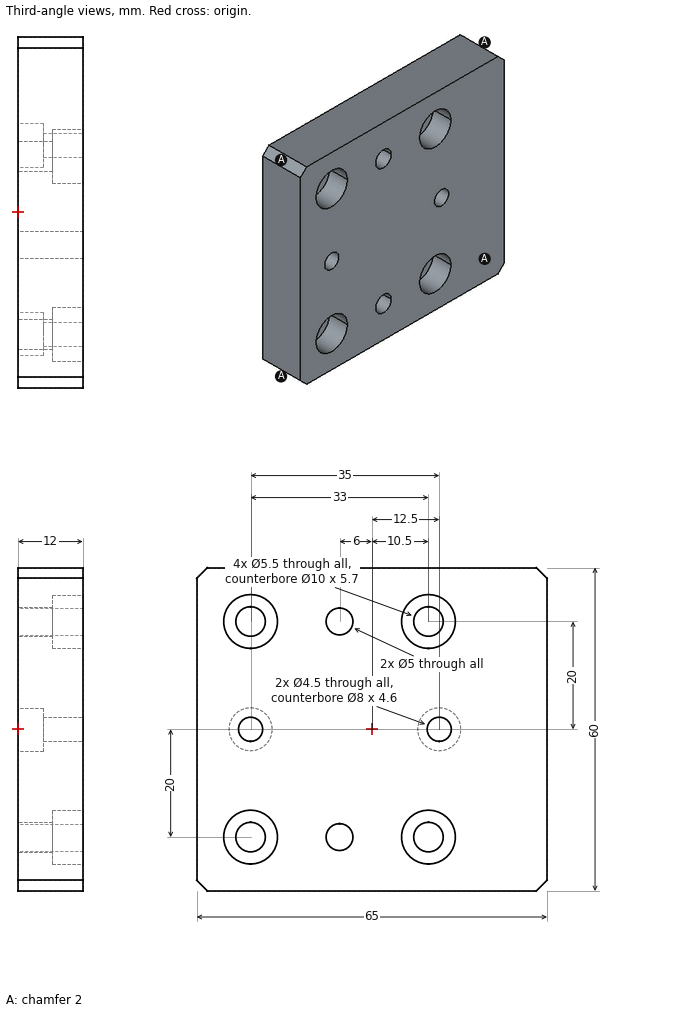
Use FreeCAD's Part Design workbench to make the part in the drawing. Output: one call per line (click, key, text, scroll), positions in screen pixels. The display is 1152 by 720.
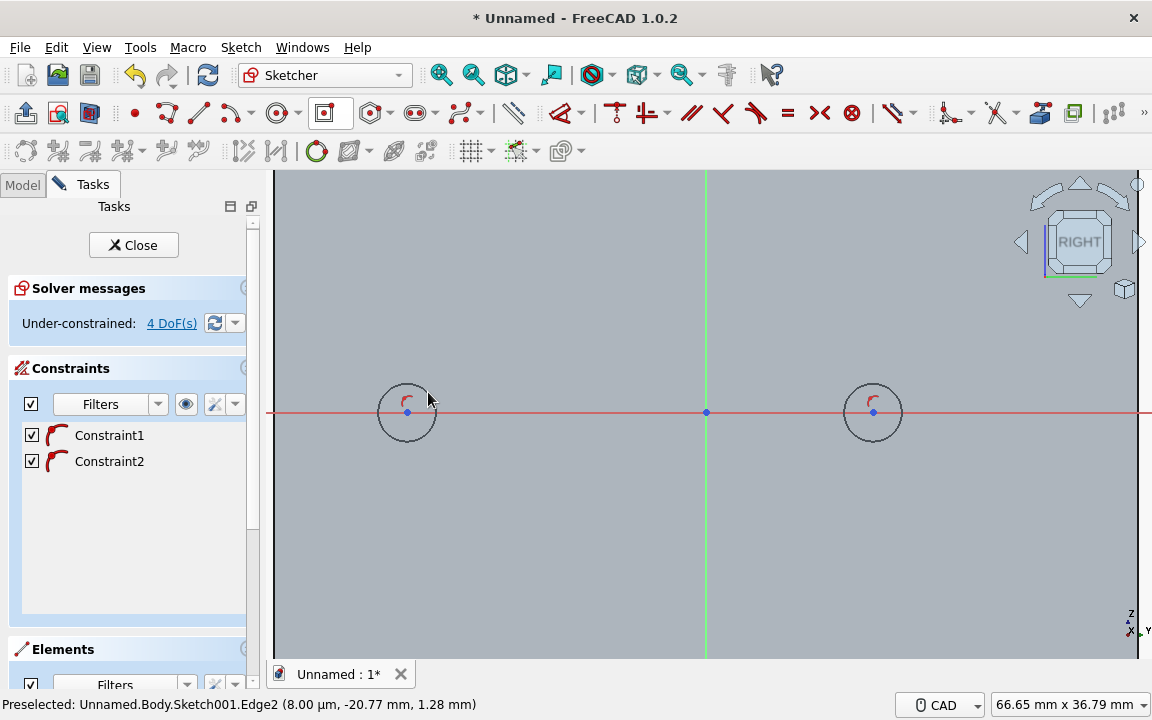
click(893, 392)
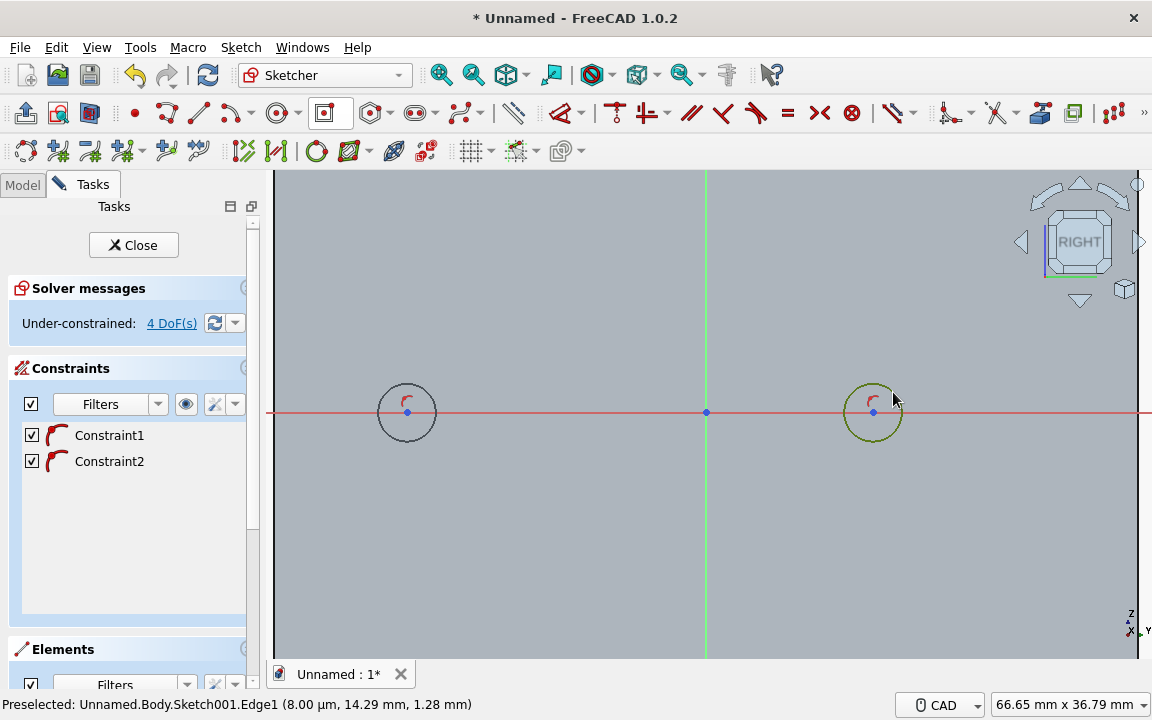
click(427, 392)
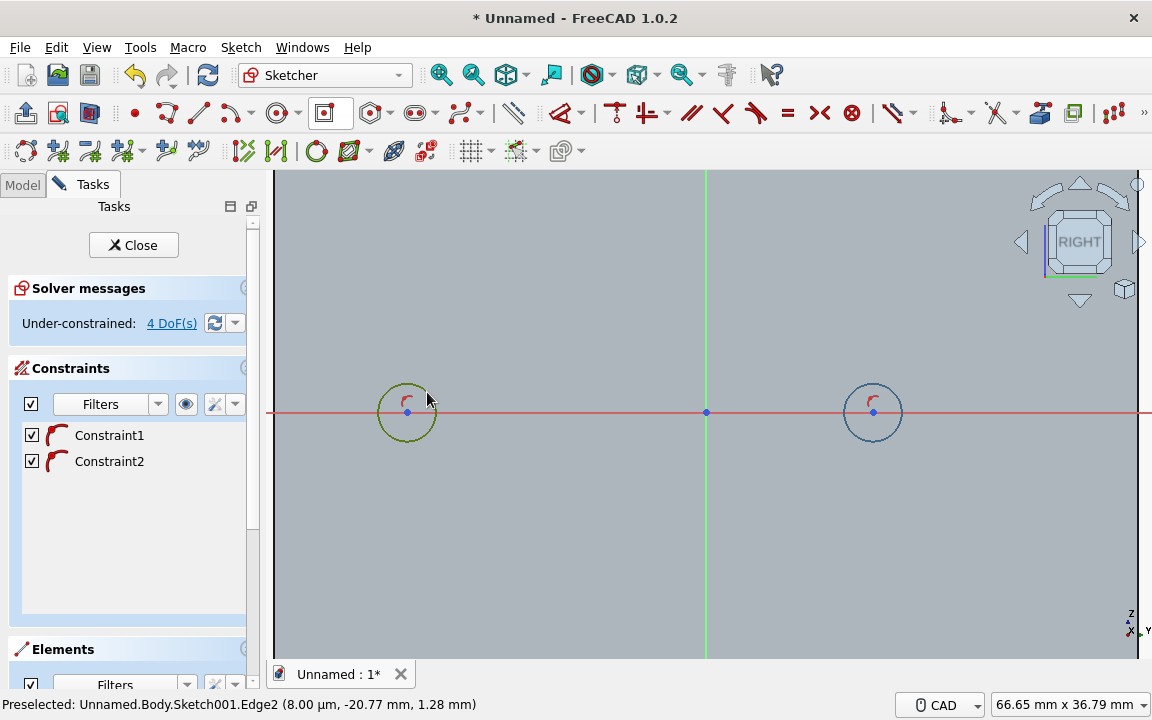
click(788, 114)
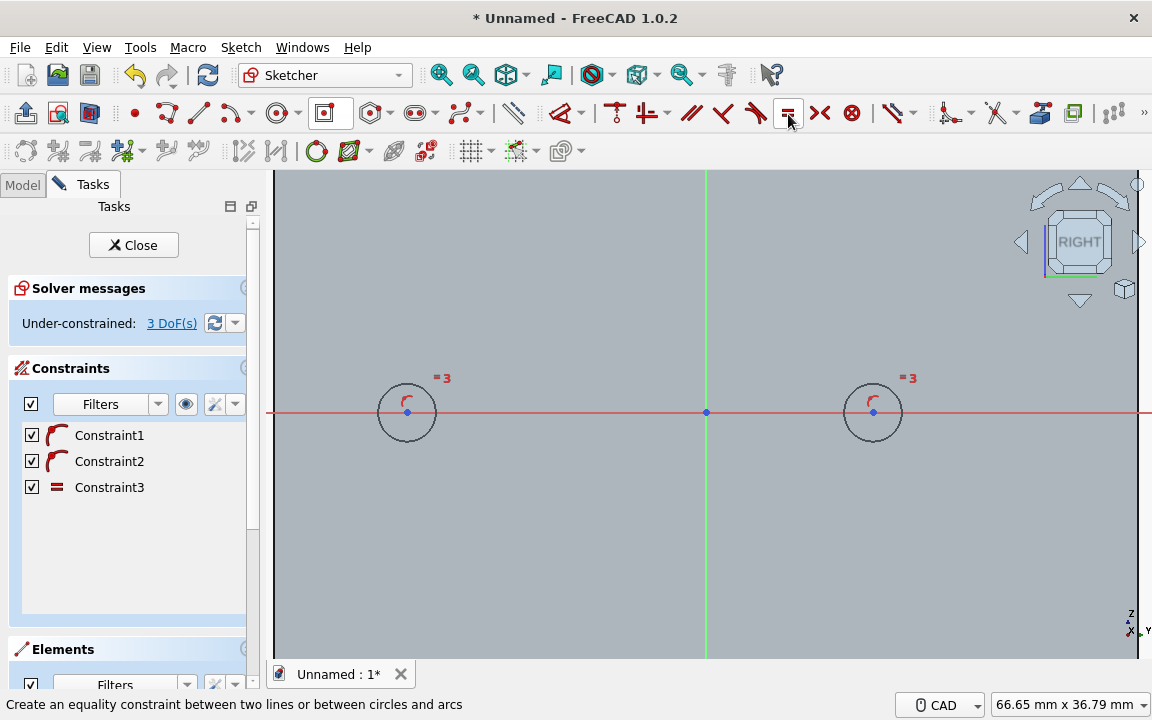
click(560, 114)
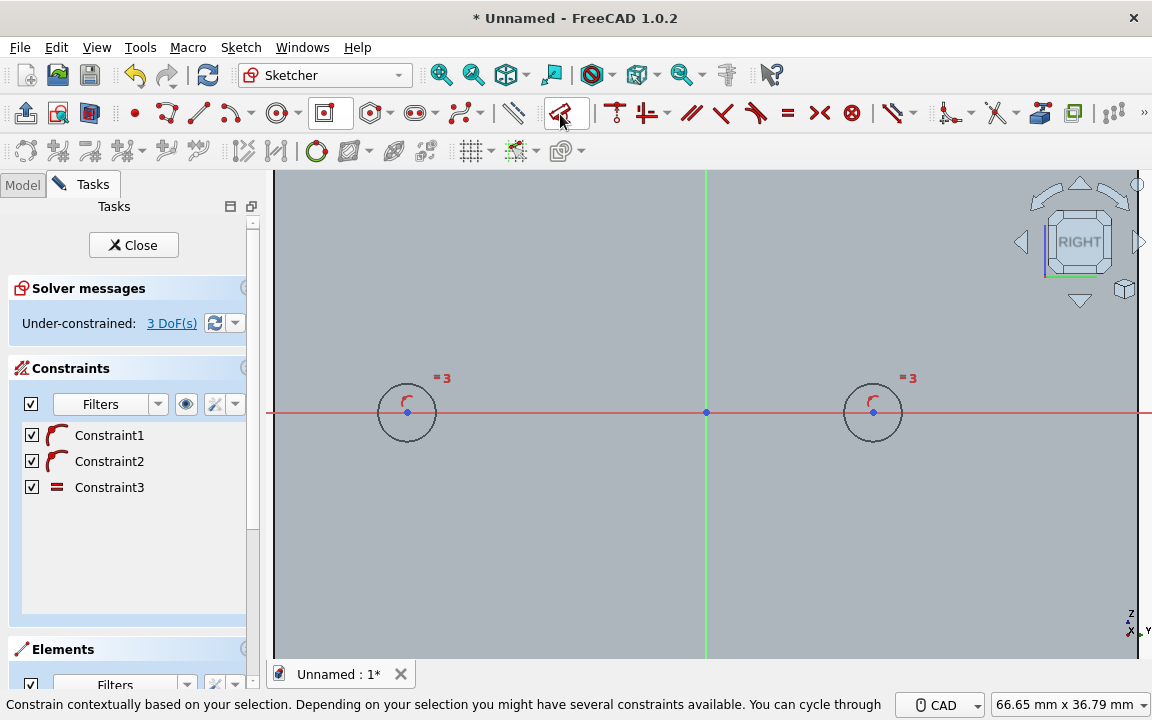
click(893, 392)
click(915, 369)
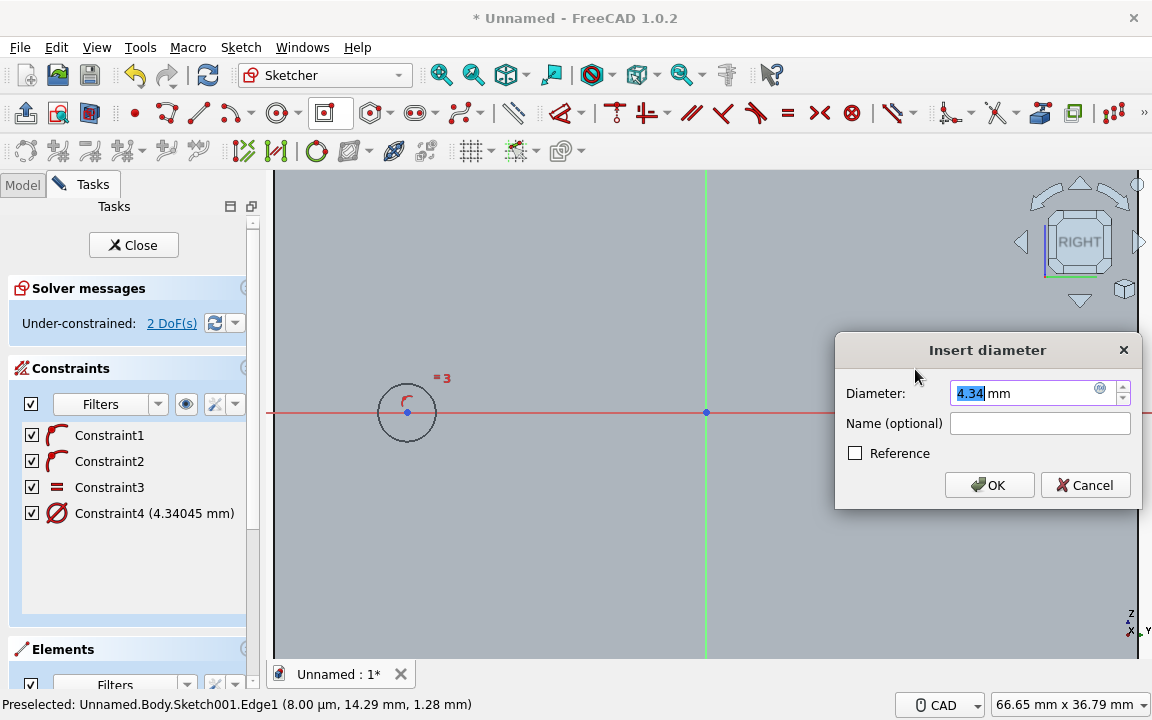
text(4.5)
key(Return)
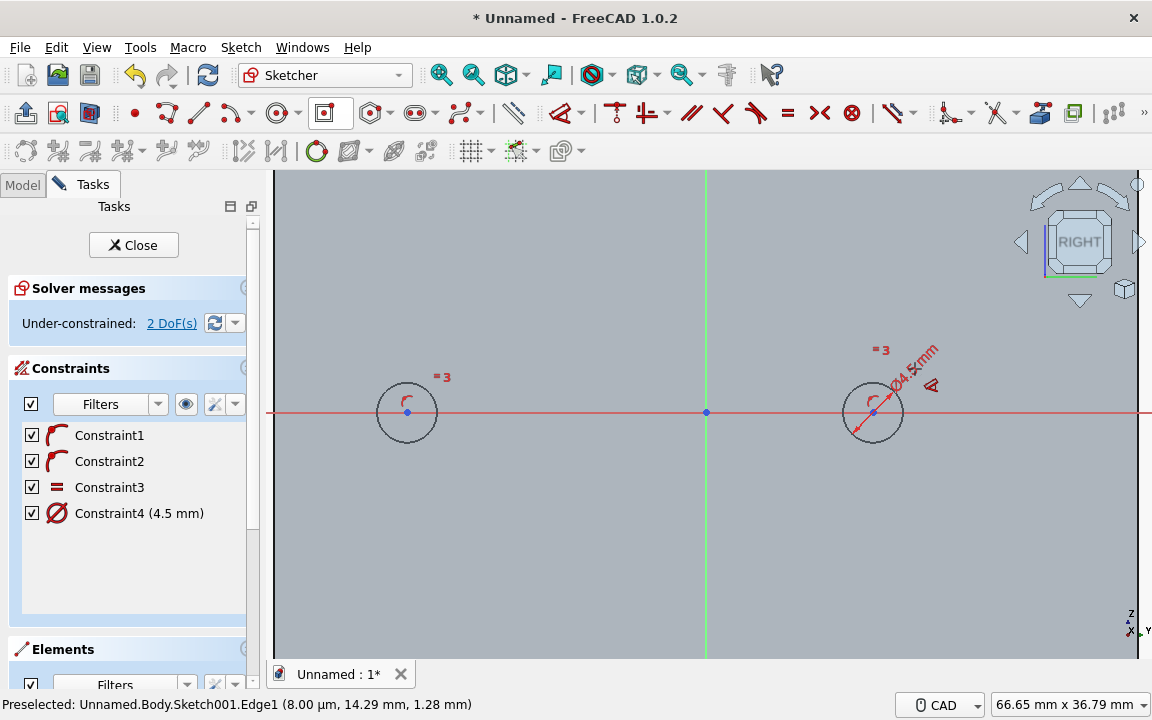
click(873, 413)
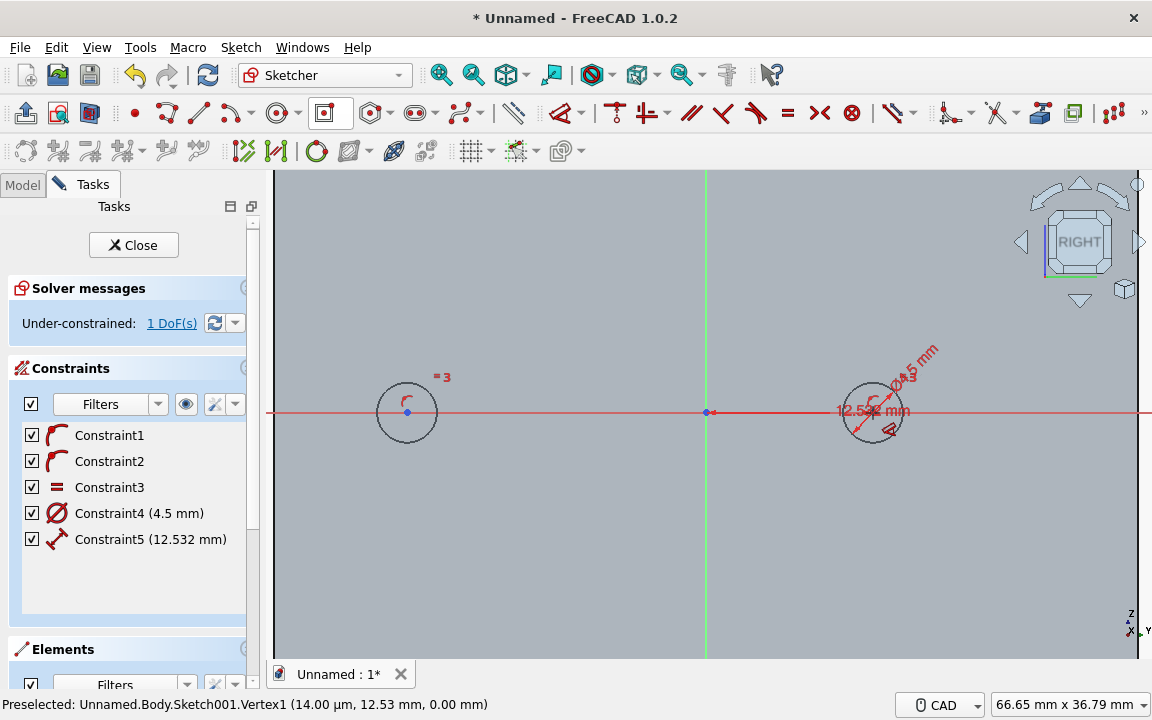
click(407, 413)
click(640, 447)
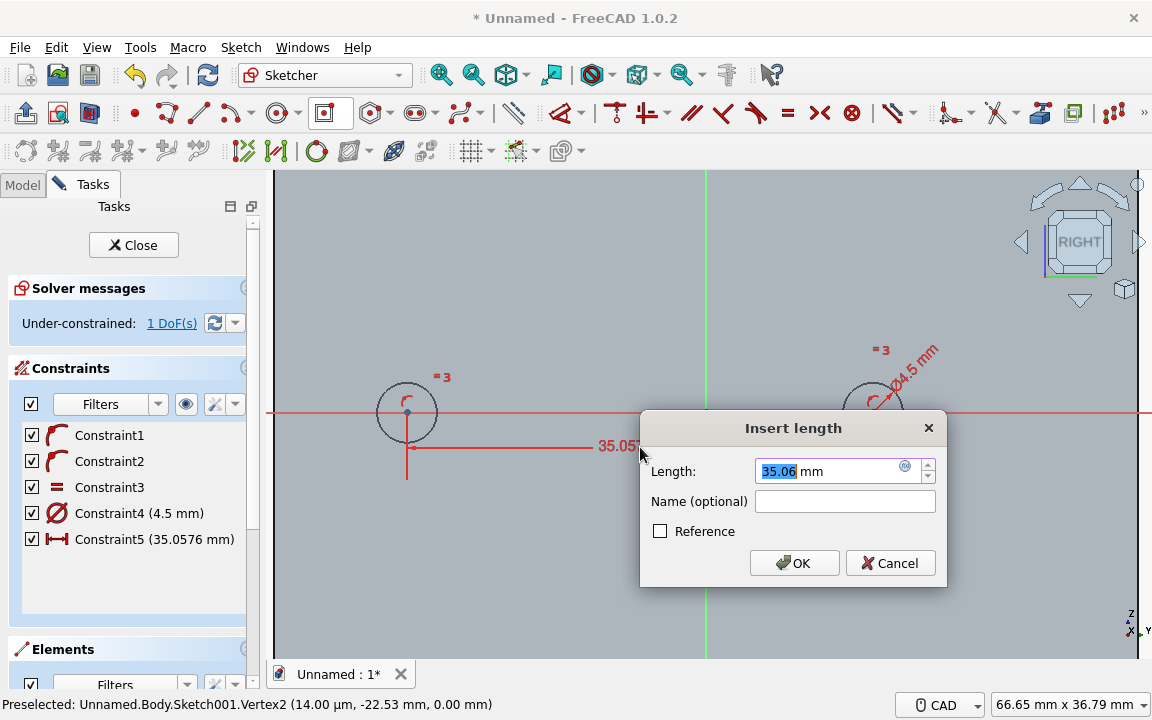
text(35)
key(Return)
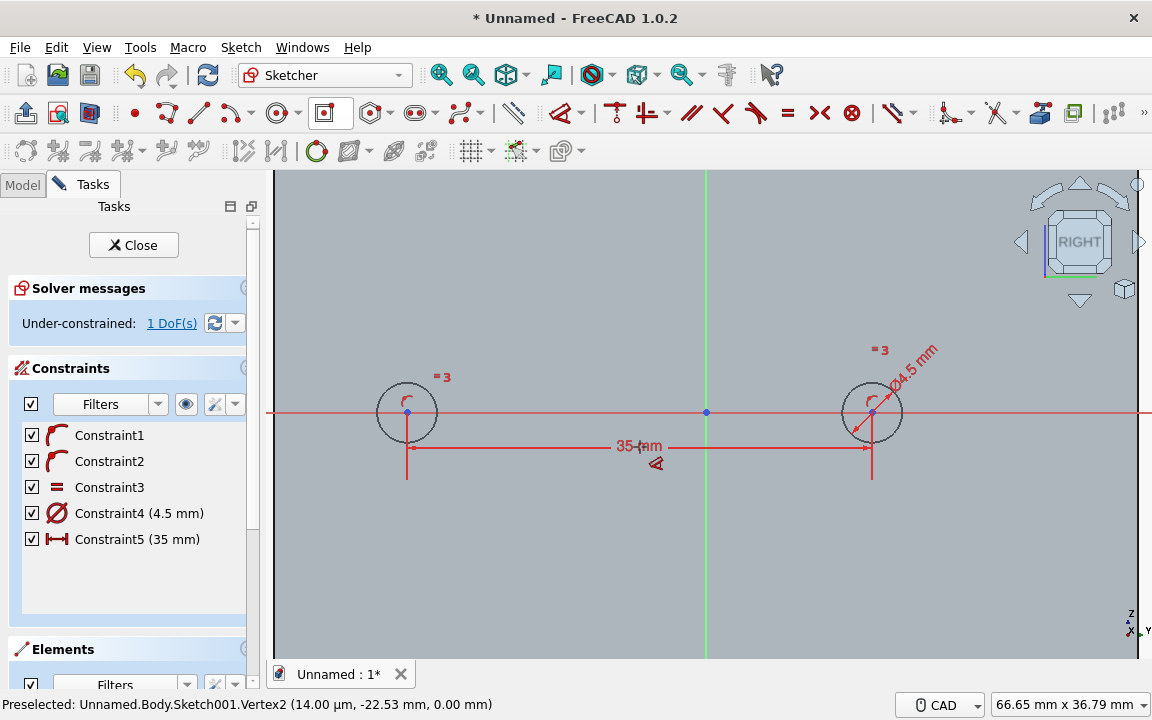
click(872, 413)
click(789, 447)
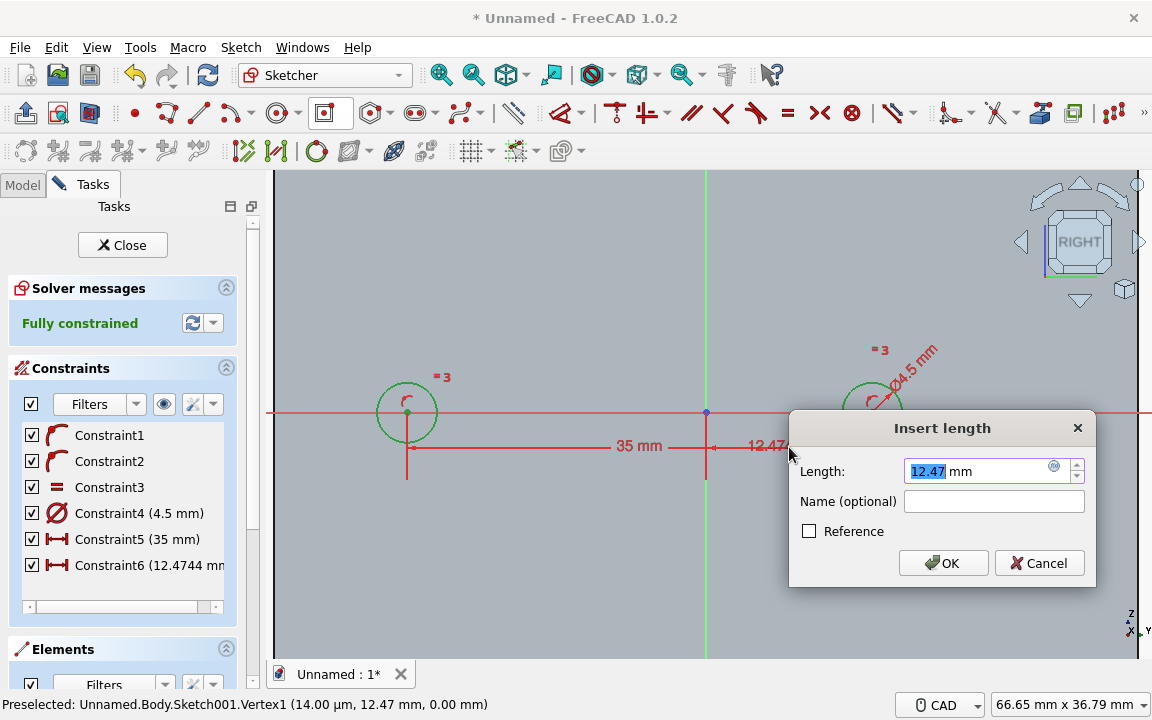
text(12.5)
key(Return)
key(Escape)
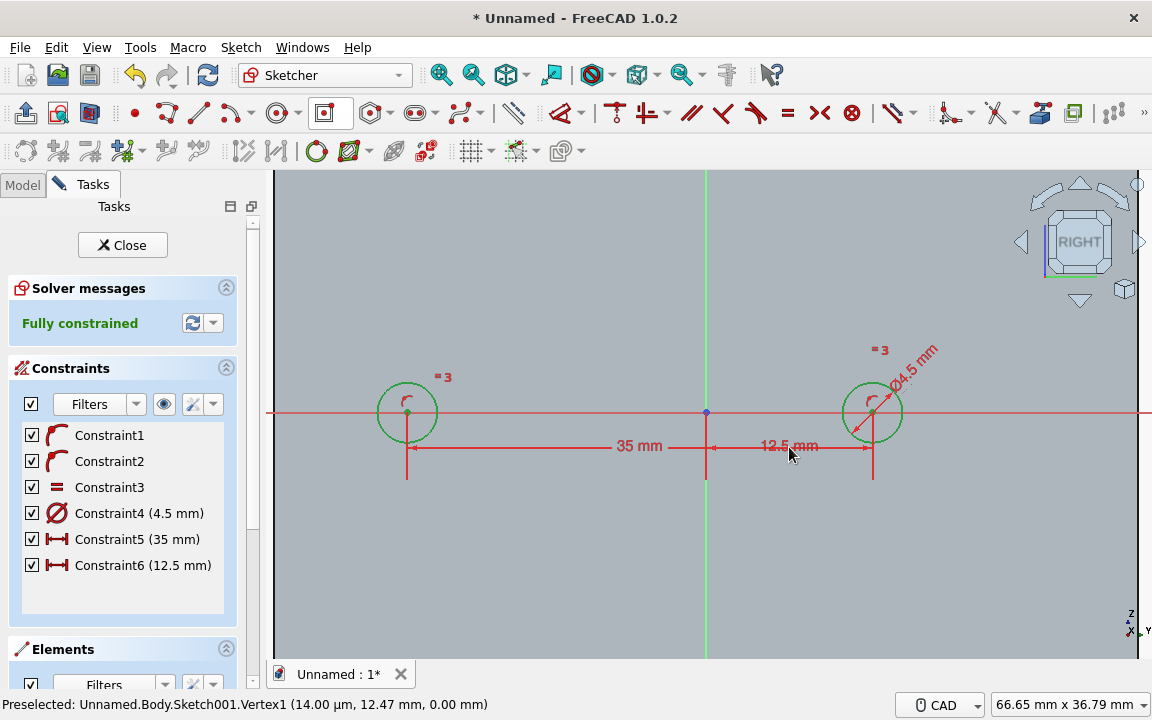
click(123, 245)